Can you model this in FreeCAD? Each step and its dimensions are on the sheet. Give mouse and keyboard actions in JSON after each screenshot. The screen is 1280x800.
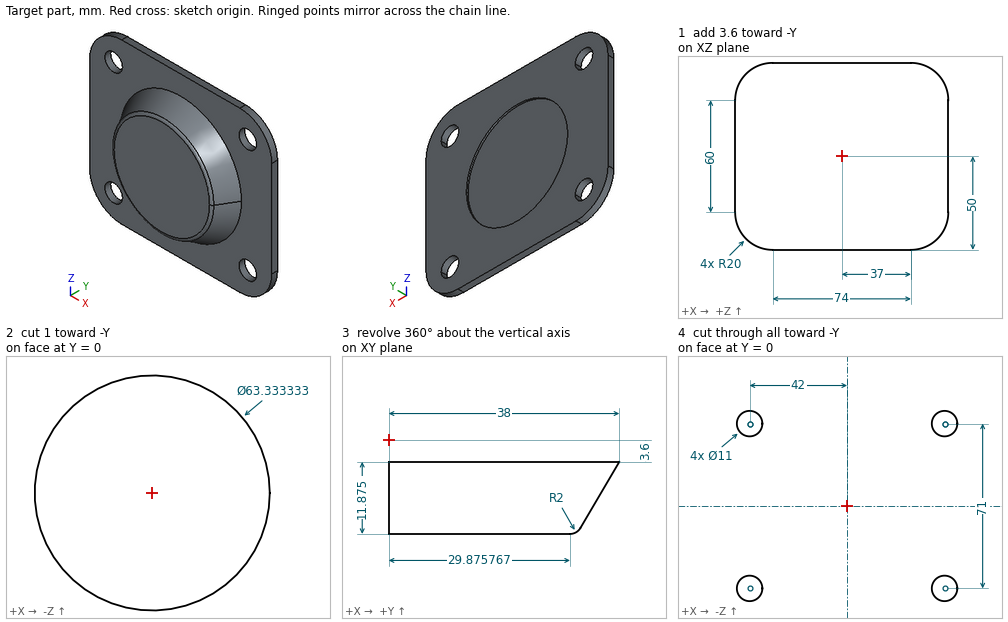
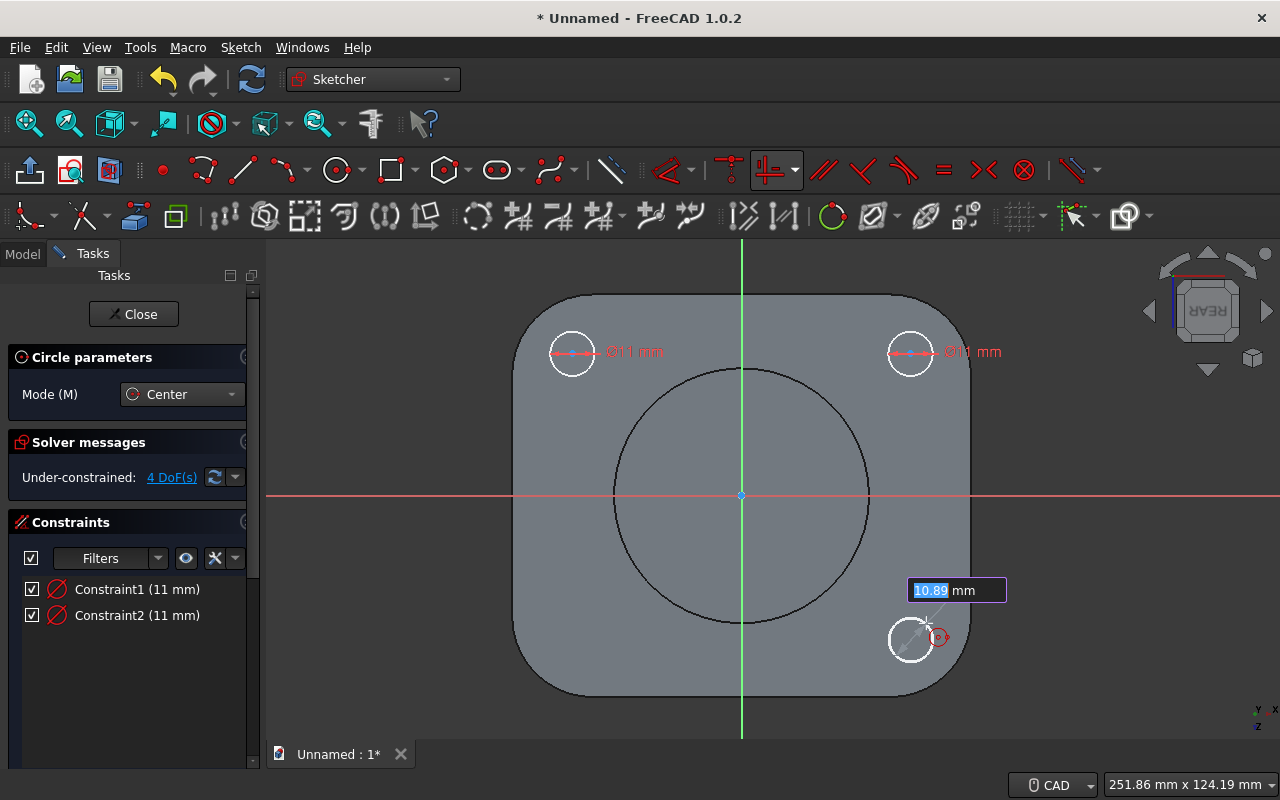
{"action": "type", "text": "11"}
{"action": "key", "text": "Return"}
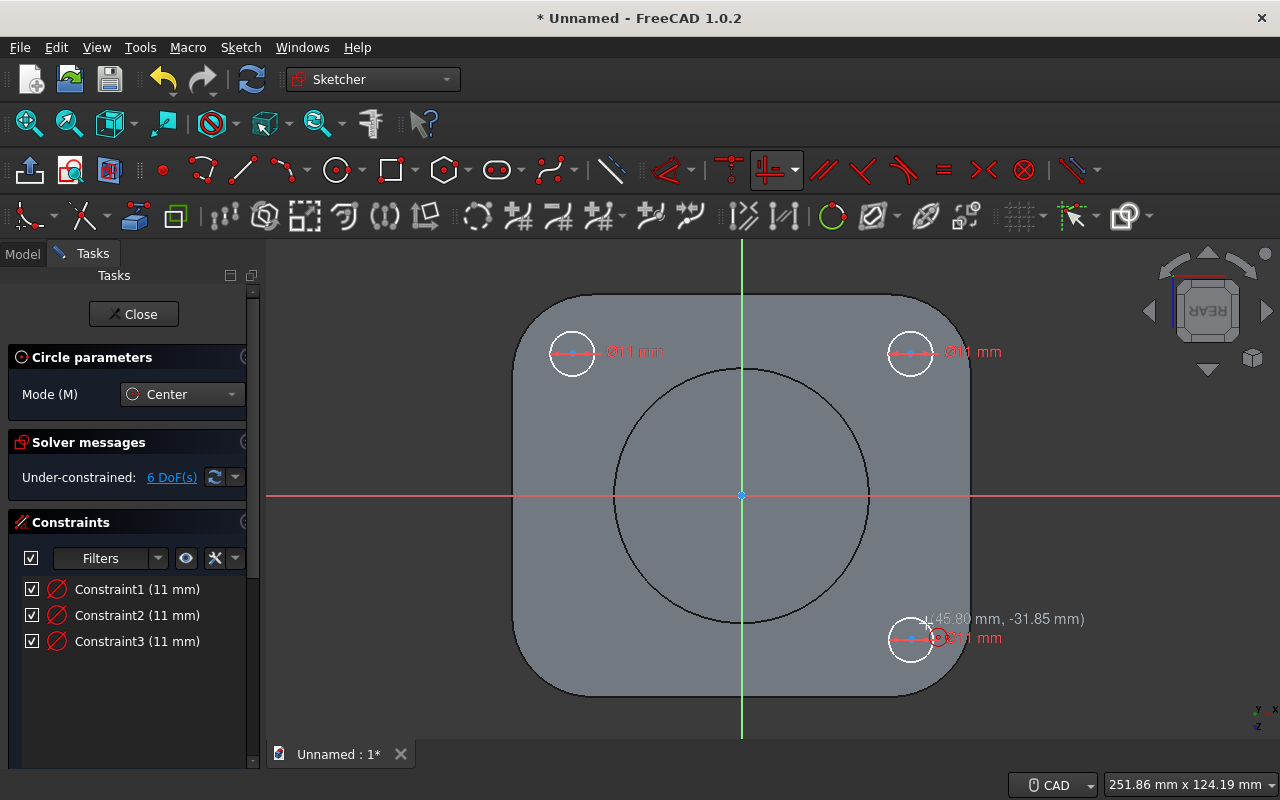
{"action": "left_click", "coordinate": [573, 639]}
{"action": "mouse_move", "coordinate": [588, 623]}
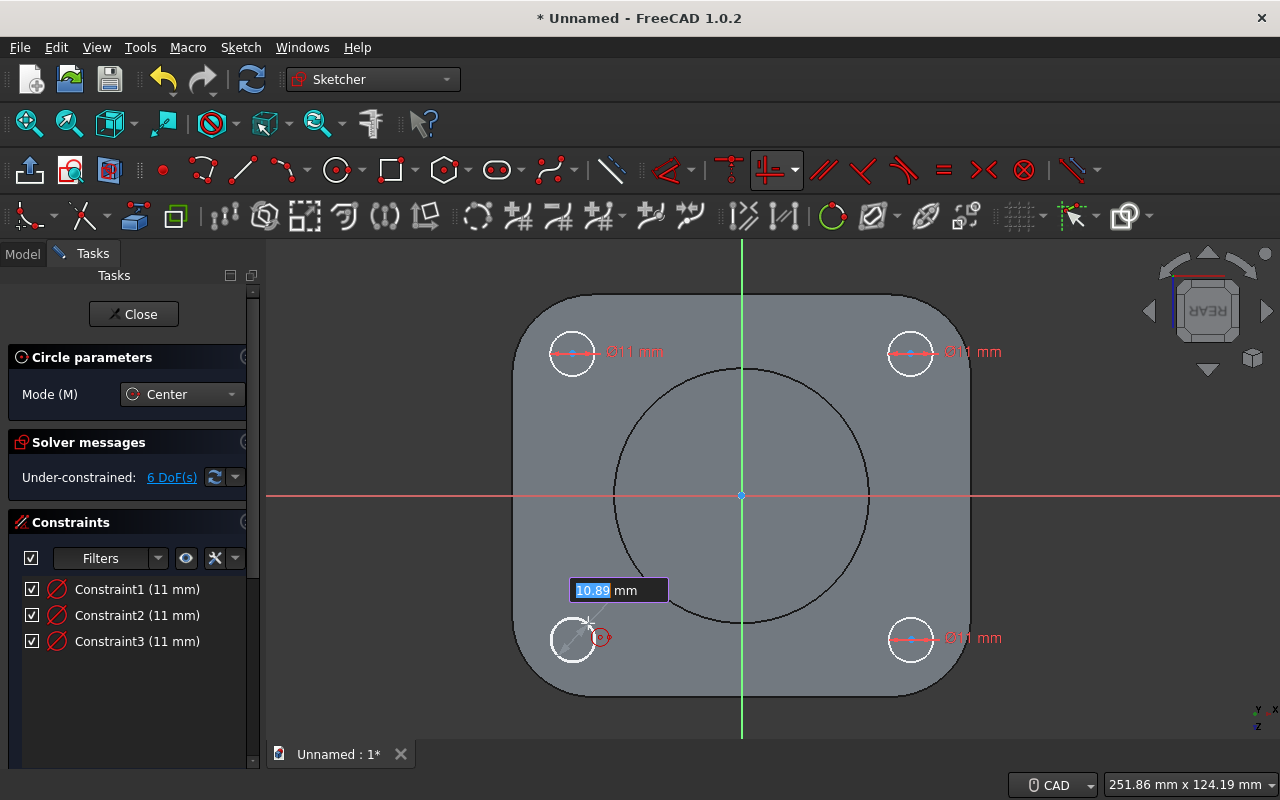
{"action": "type", "text": "11"}
{"action": "key", "text": "Return"}
{"action": "key", "text": "Escape"}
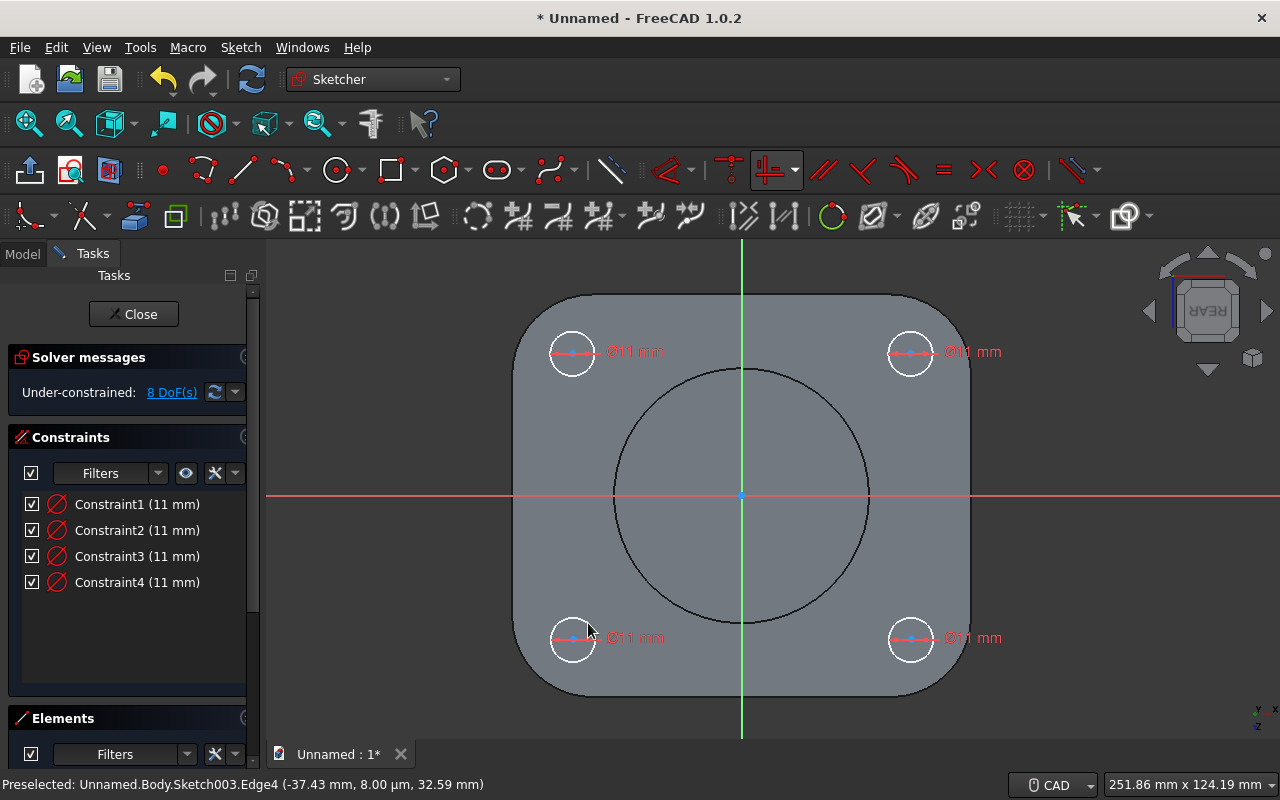
{"action": "left_click", "coordinate": [572, 354]}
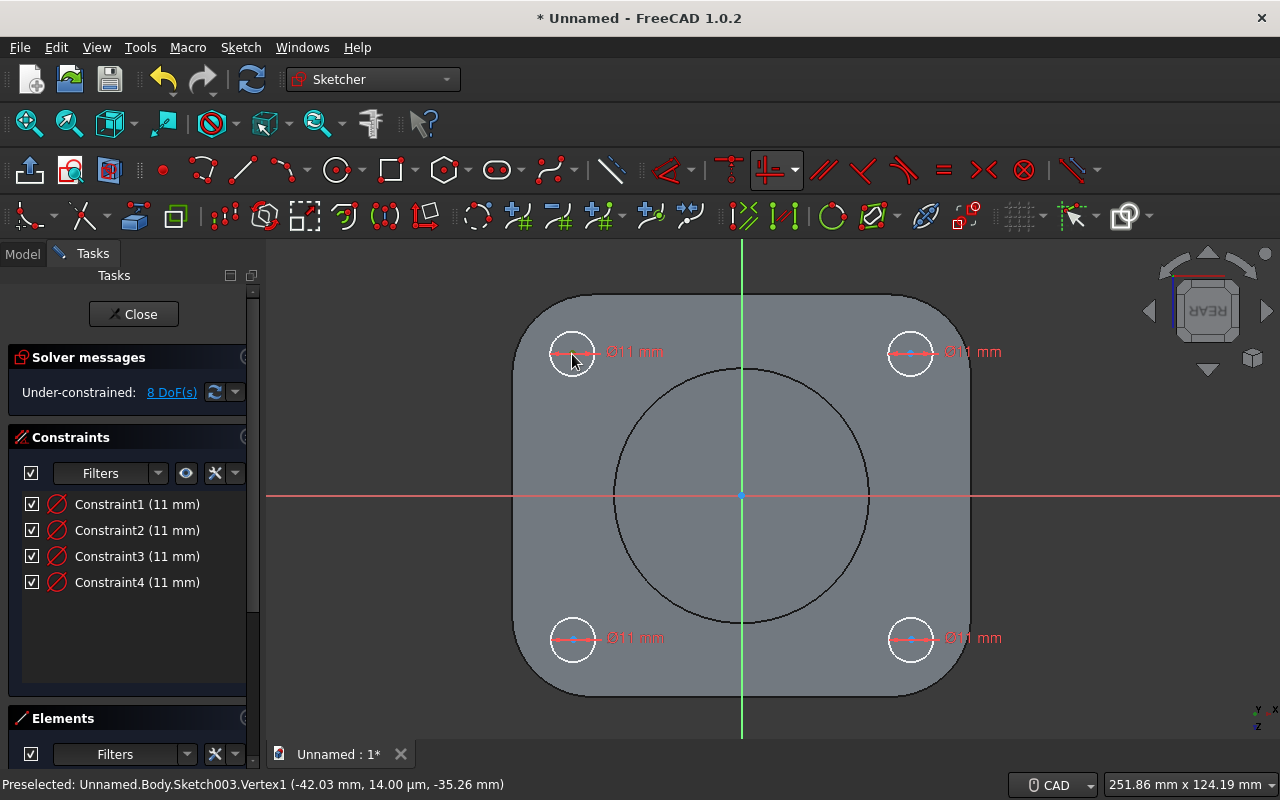
{"action": "left_click", "coordinate": [911, 354]}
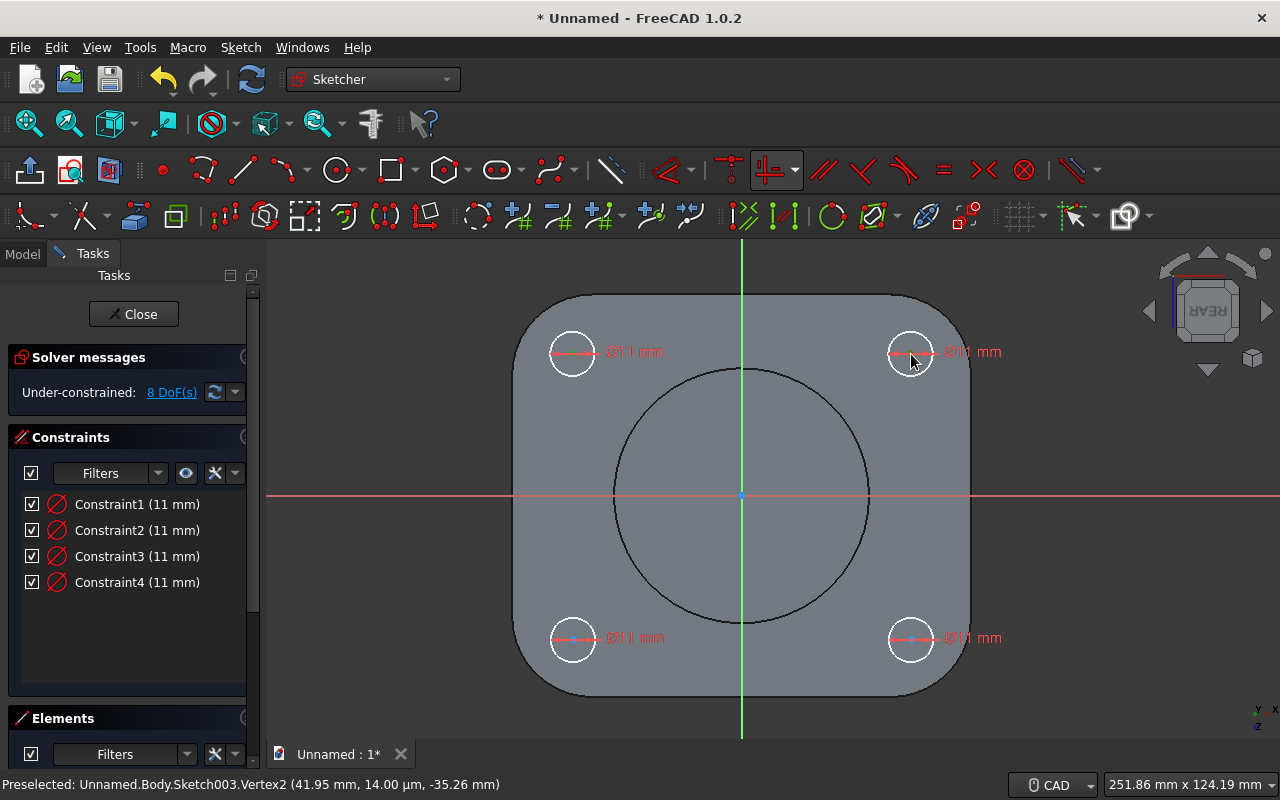
{"action": "left_click", "coordinate": [742, 679]}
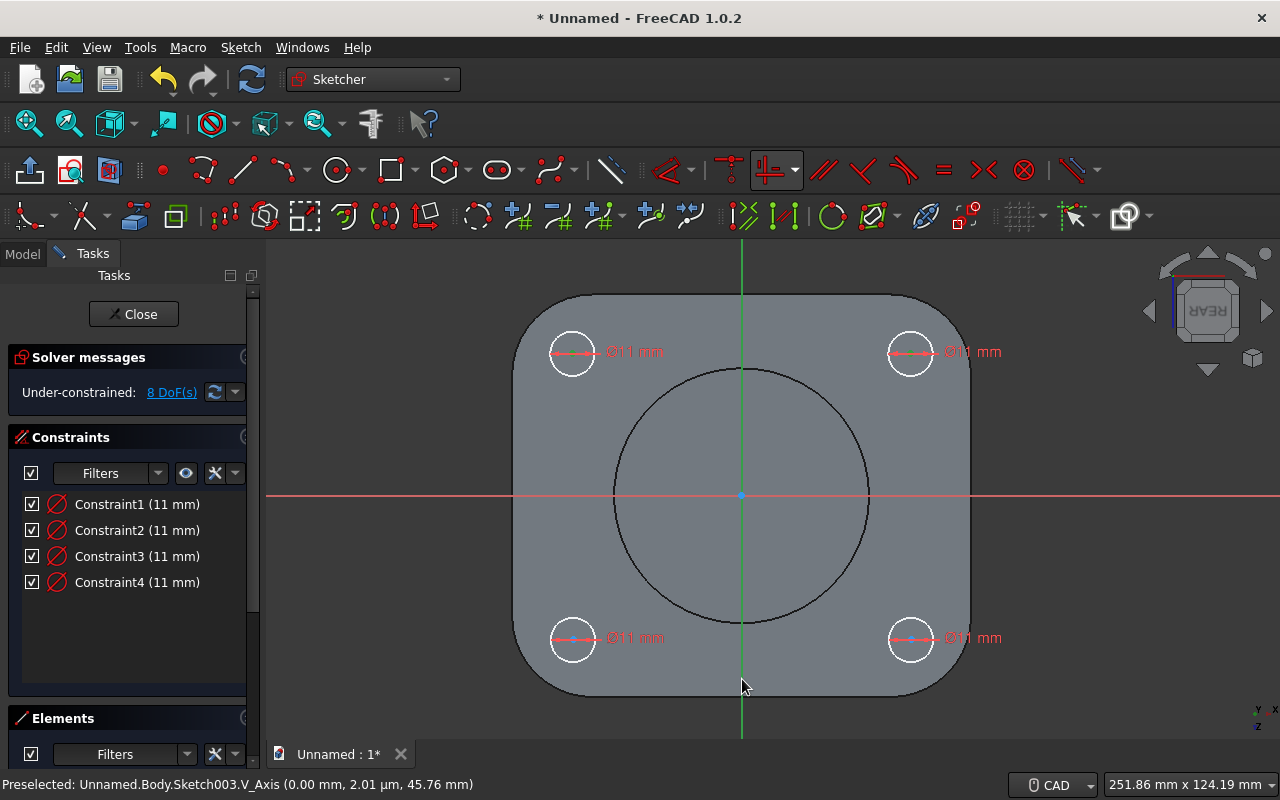
{"action": "left_click", "coordinate": [984, 170]}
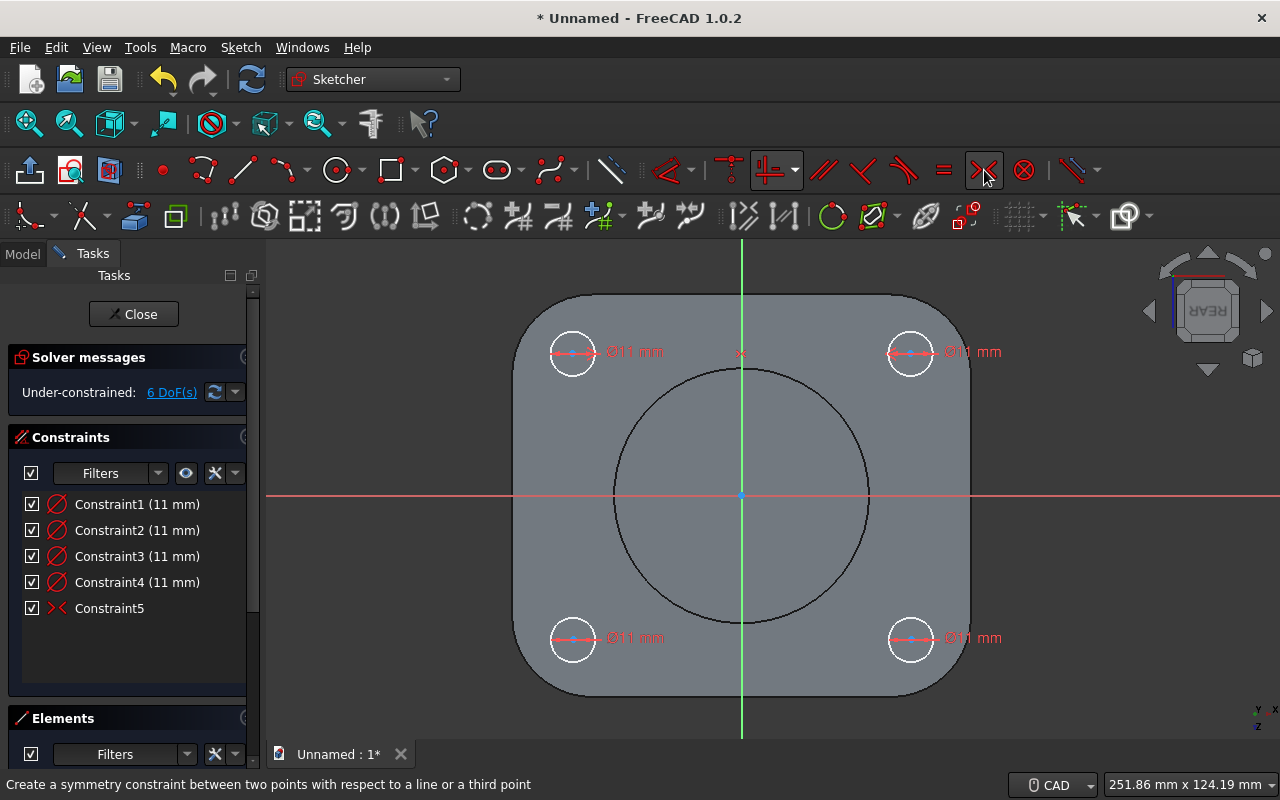
{"action": "left_click", "coordinate": [911, 354]}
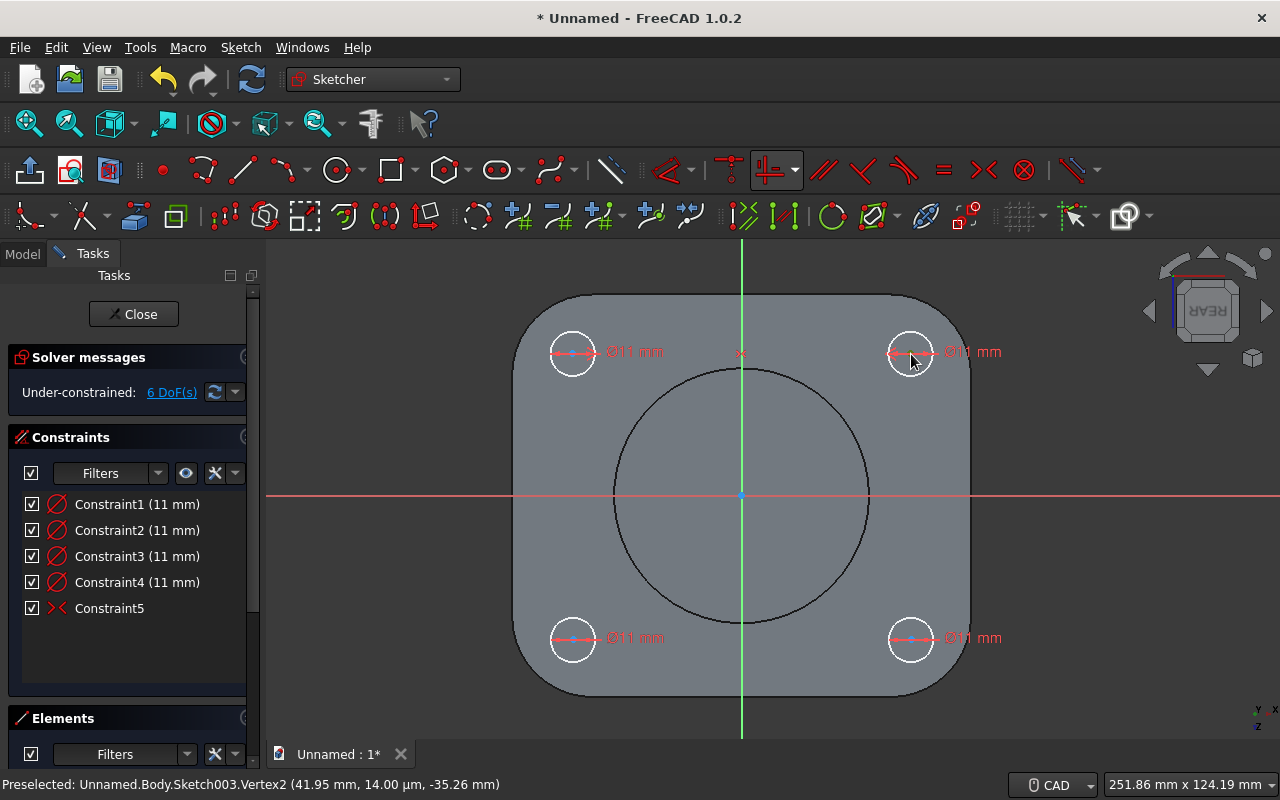
{"action": "left_click", "coordinate": [911, 640]}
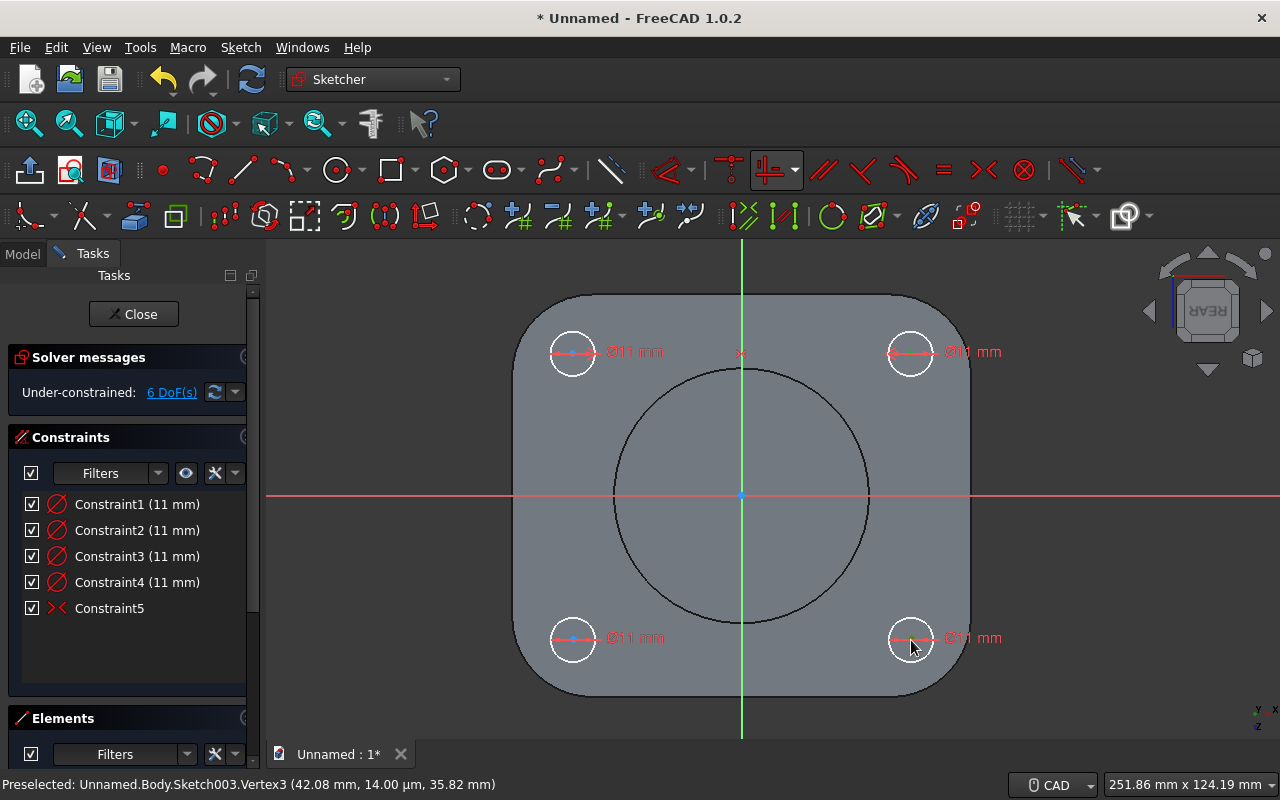
{"action": "left_click", "coordinate": [353, 496]}